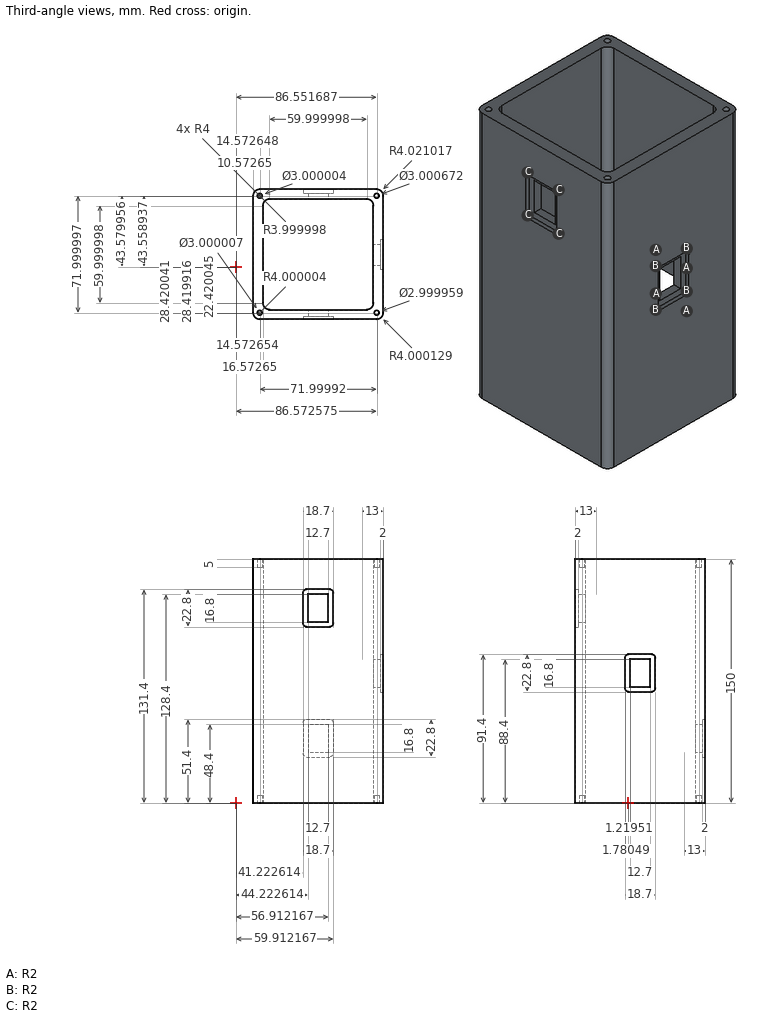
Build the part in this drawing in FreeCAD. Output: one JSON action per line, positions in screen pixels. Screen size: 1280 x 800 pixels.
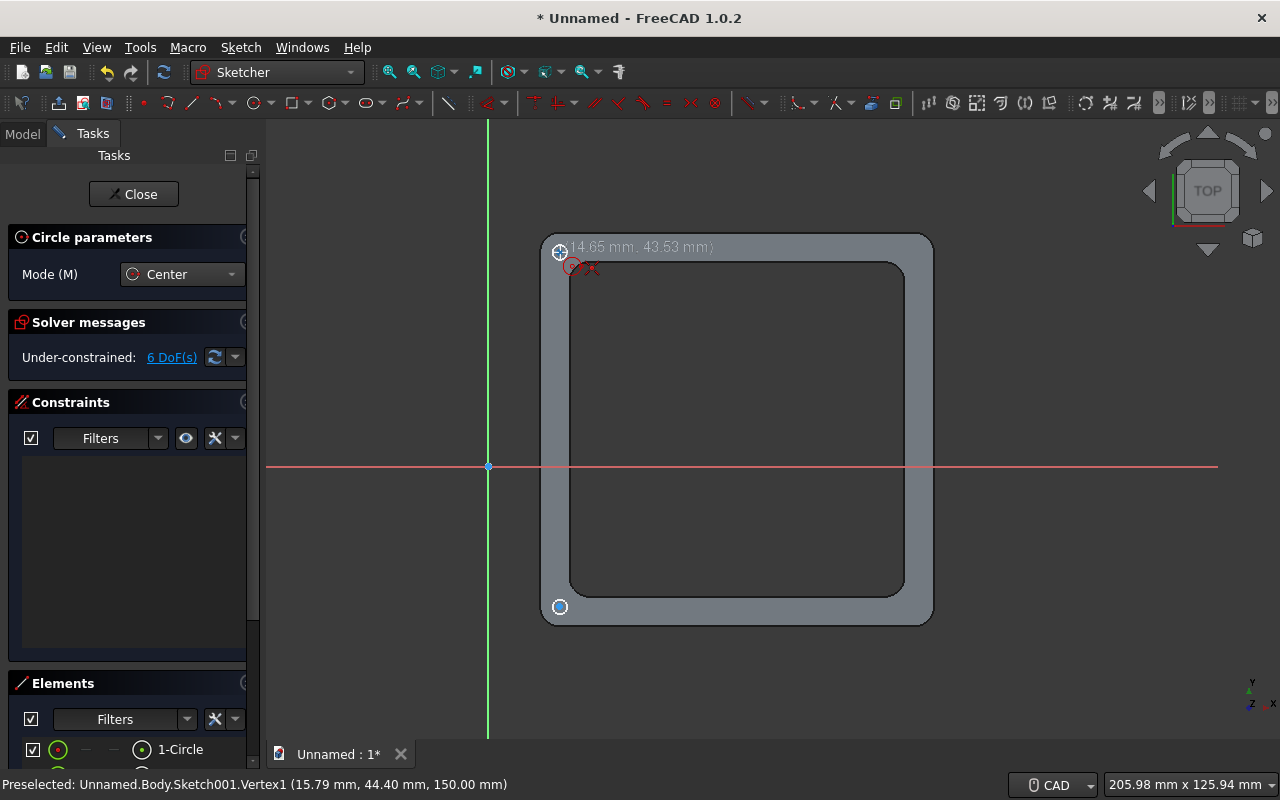
{"action": "scroll", "coordinate": [914, 252], "scroll_direction": "up", "scroll_amount": 6}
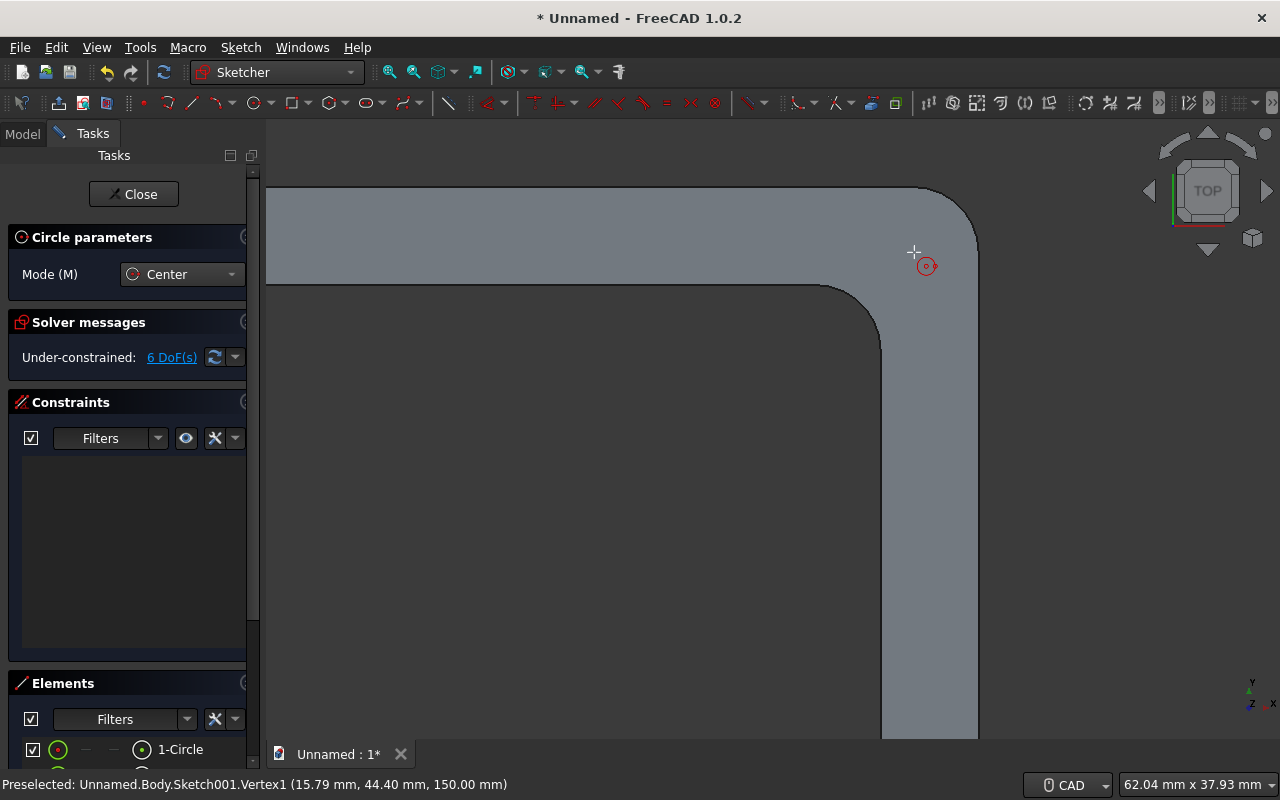
{"action": "left_click", "coordinate": [913, 253]}
{"action": "left_click", "coordinate": [930, 235]}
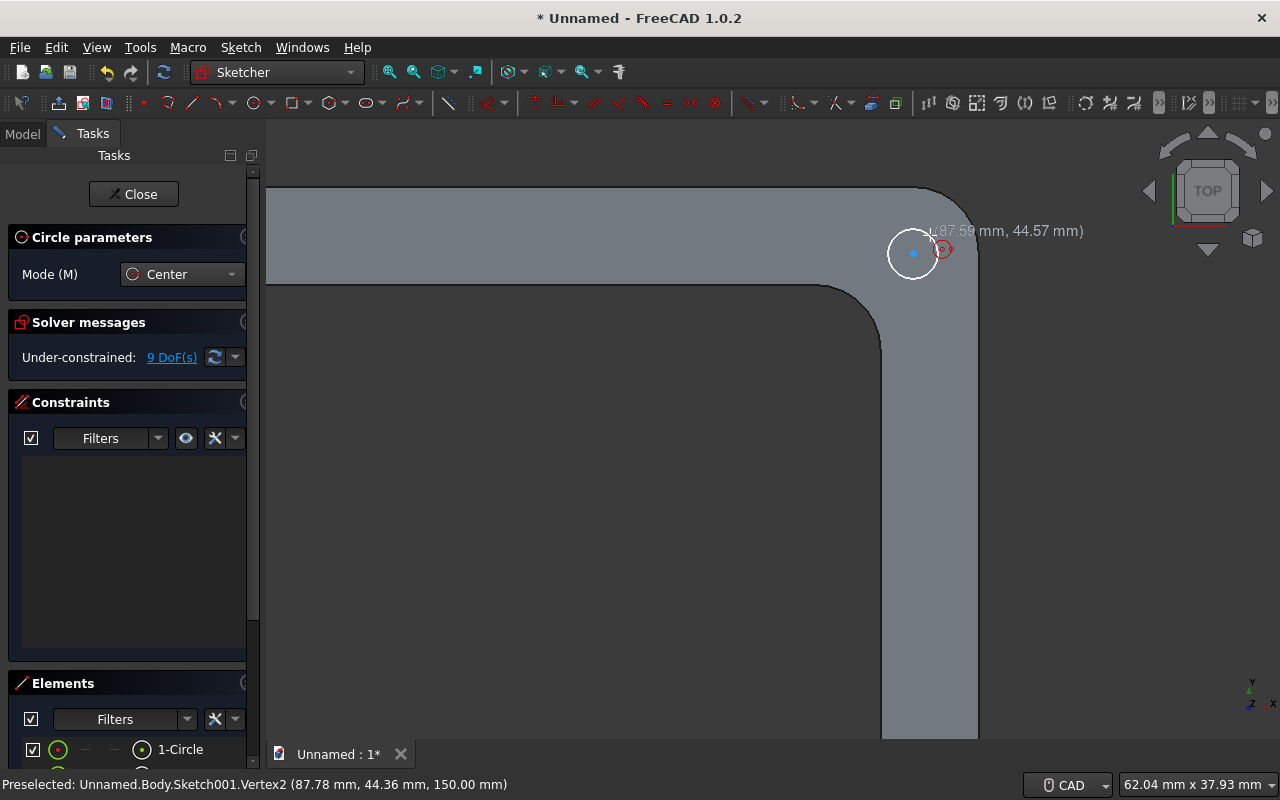
{"action": "scroll", "coordinate": [914, 252], "scroll_direction": "down", "scroll_amount": 6}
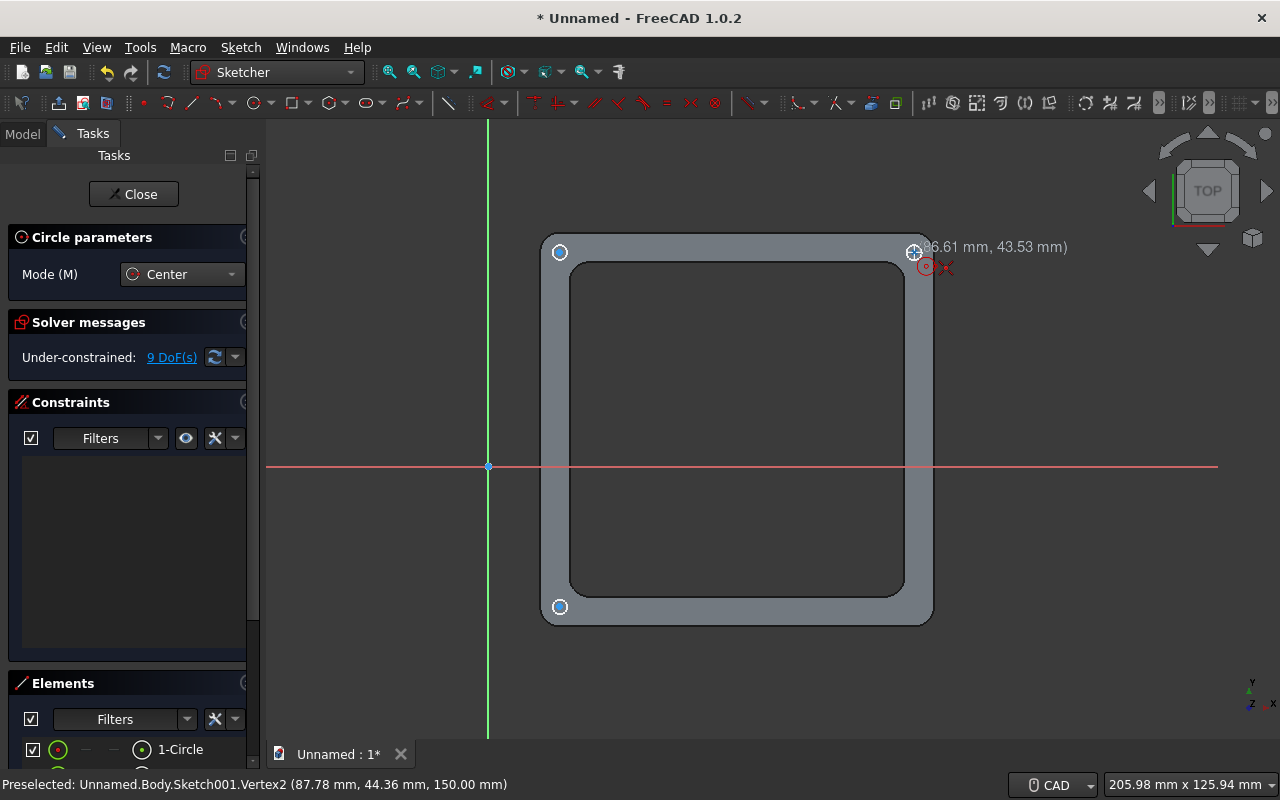
{"action": "scroll", "coordinate": [914, 607], "scroll_direction": "up", "scroll_amount": 6}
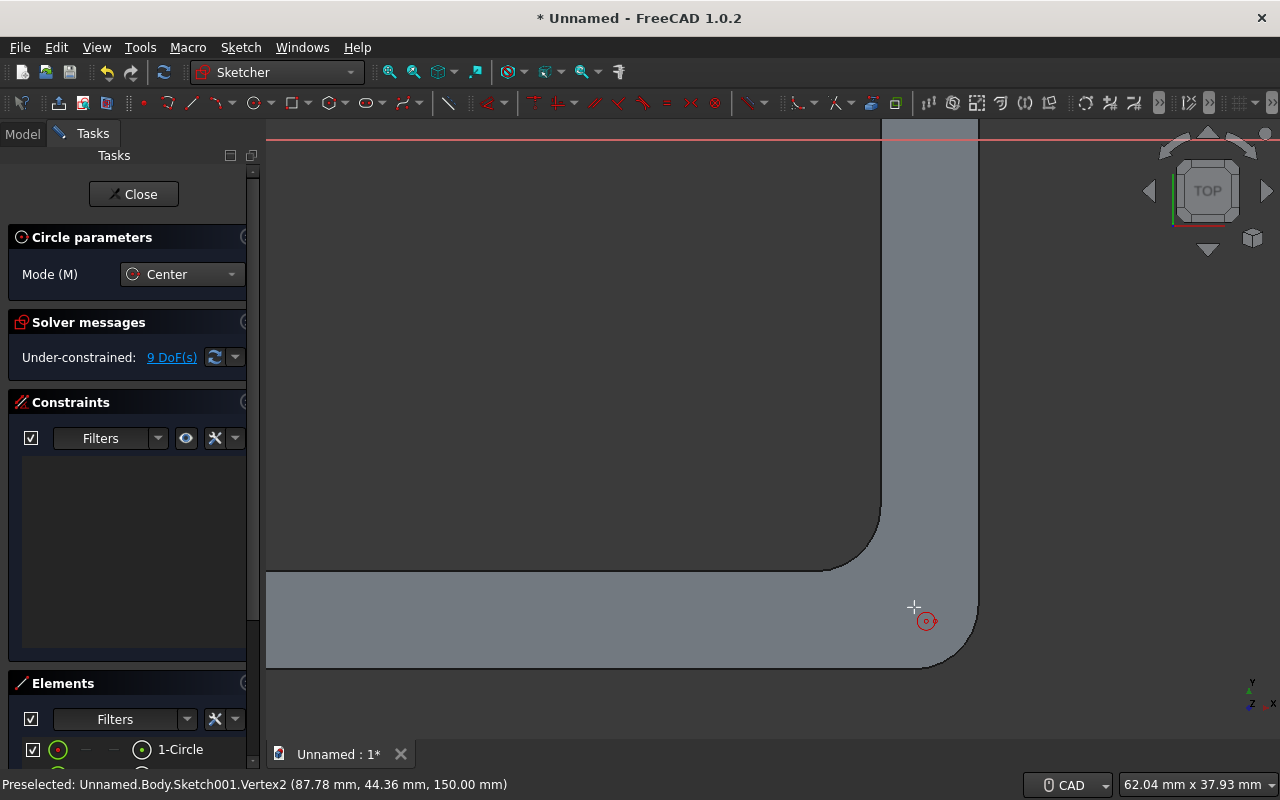
{"action": "left_click", "coordinate": [913, 604]}
{"action": "left_click", "coordinate": [931, 587]}
{"action": "key", "text": "Escape"}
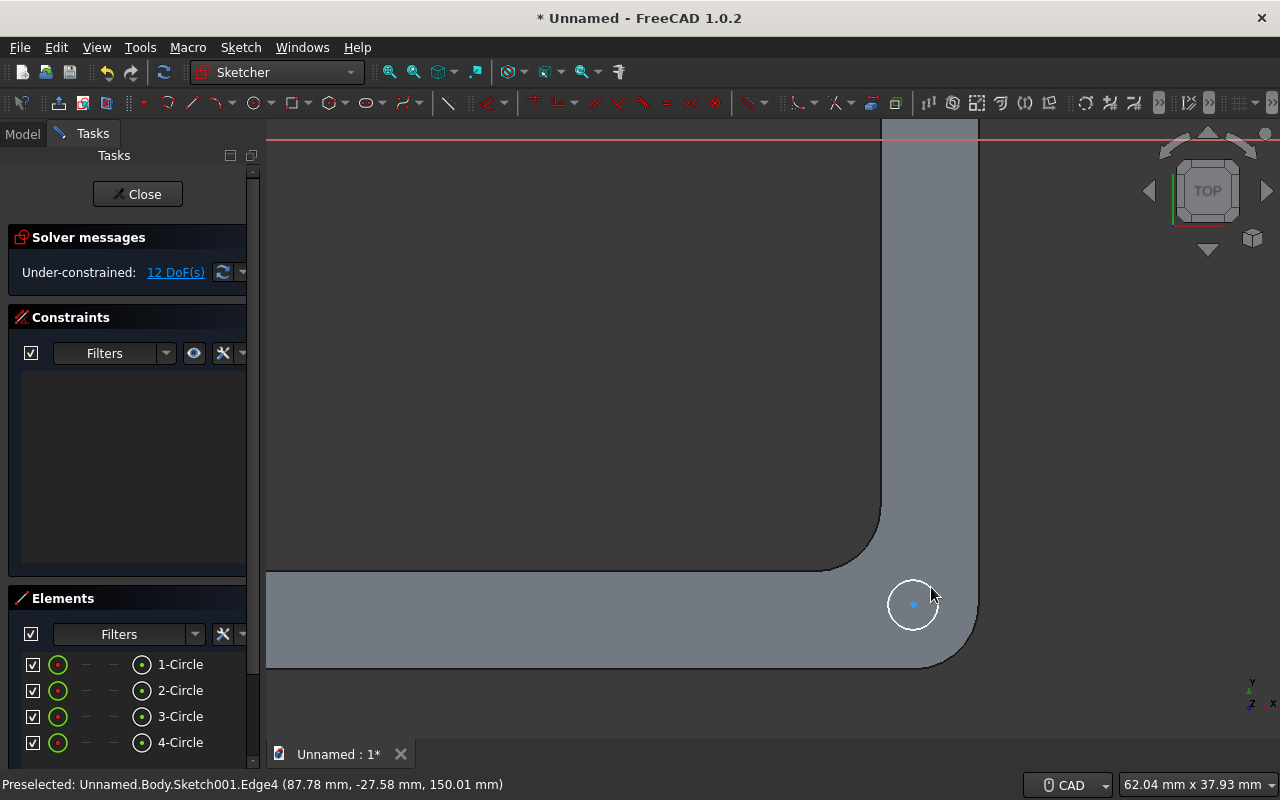
{"action": "left_click", "coordinate": [488, 104]}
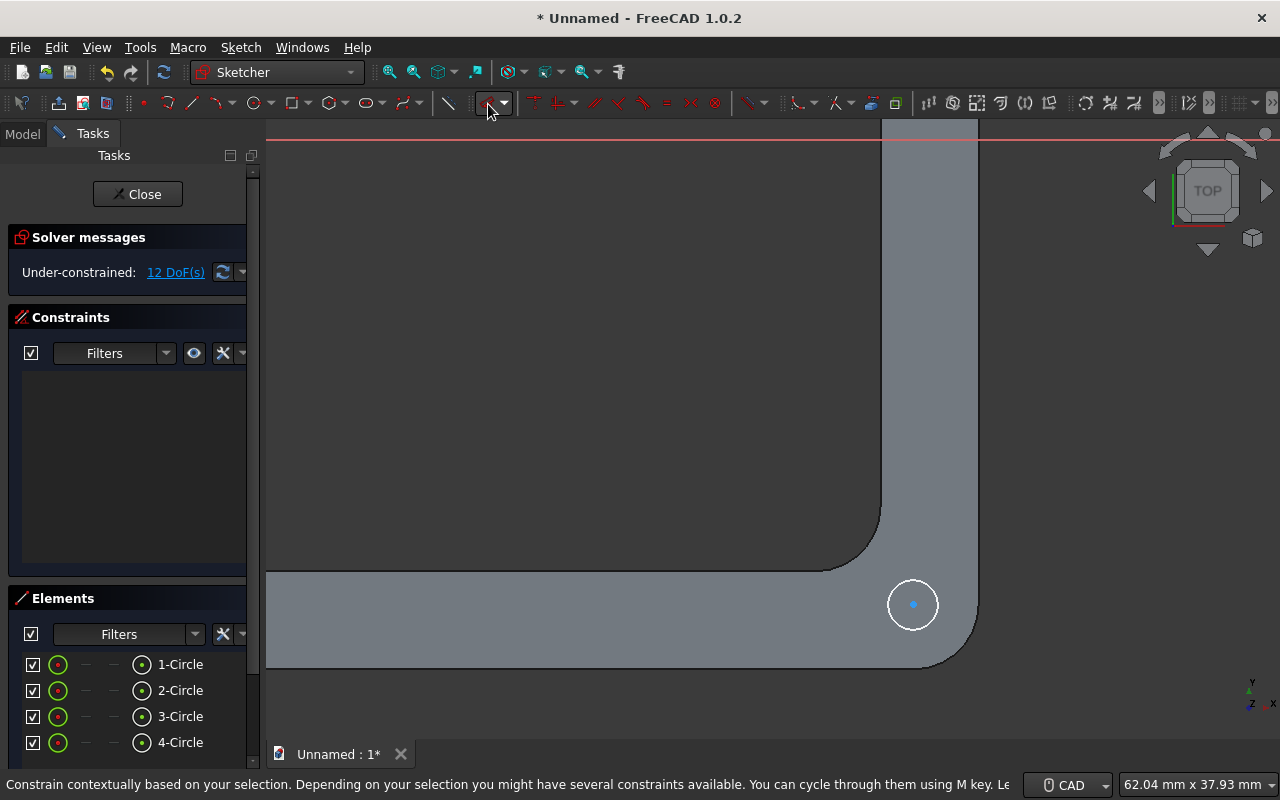
{"action": "scroll", "coordinate": [914, 607], "scroll_direction": "down", "scroll_amount": 6}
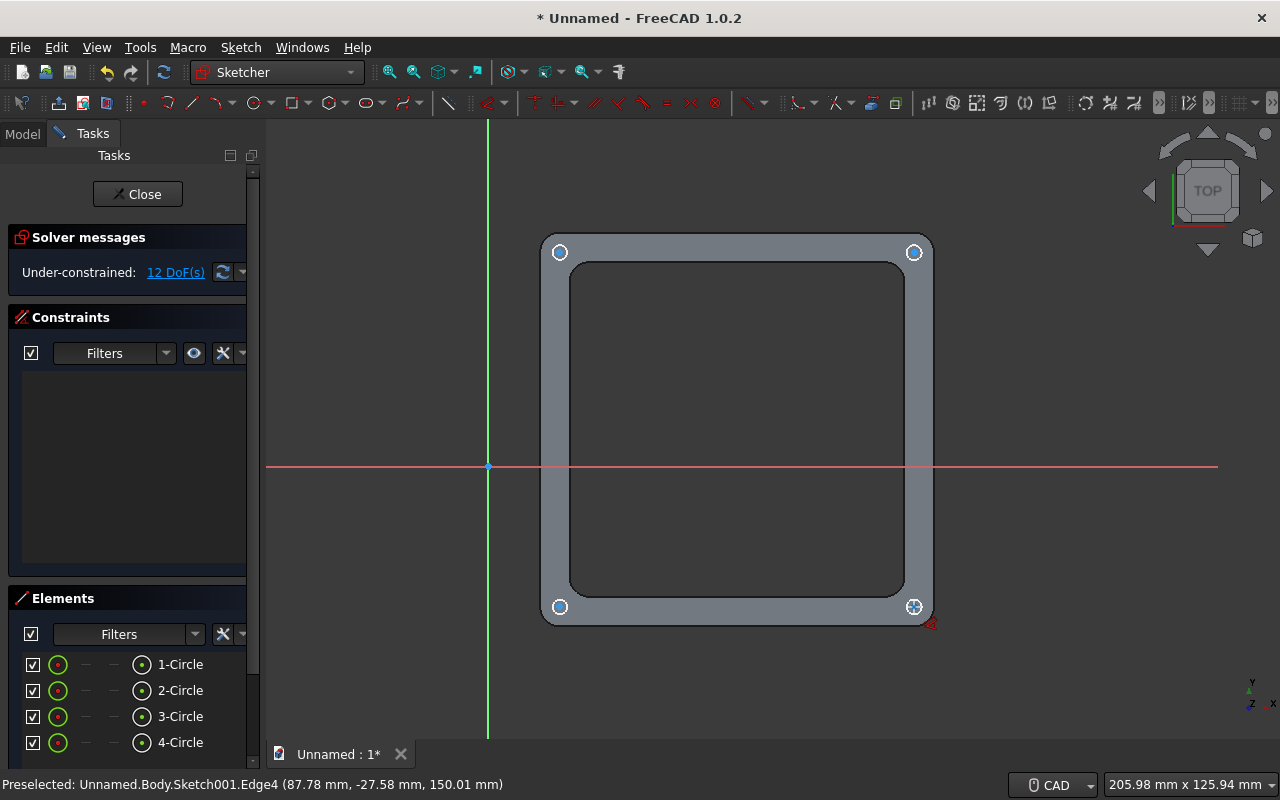
{"action": "scroll", "coordinate": [565, 602], "scroll_direction": "up", "scroll_amount": 5}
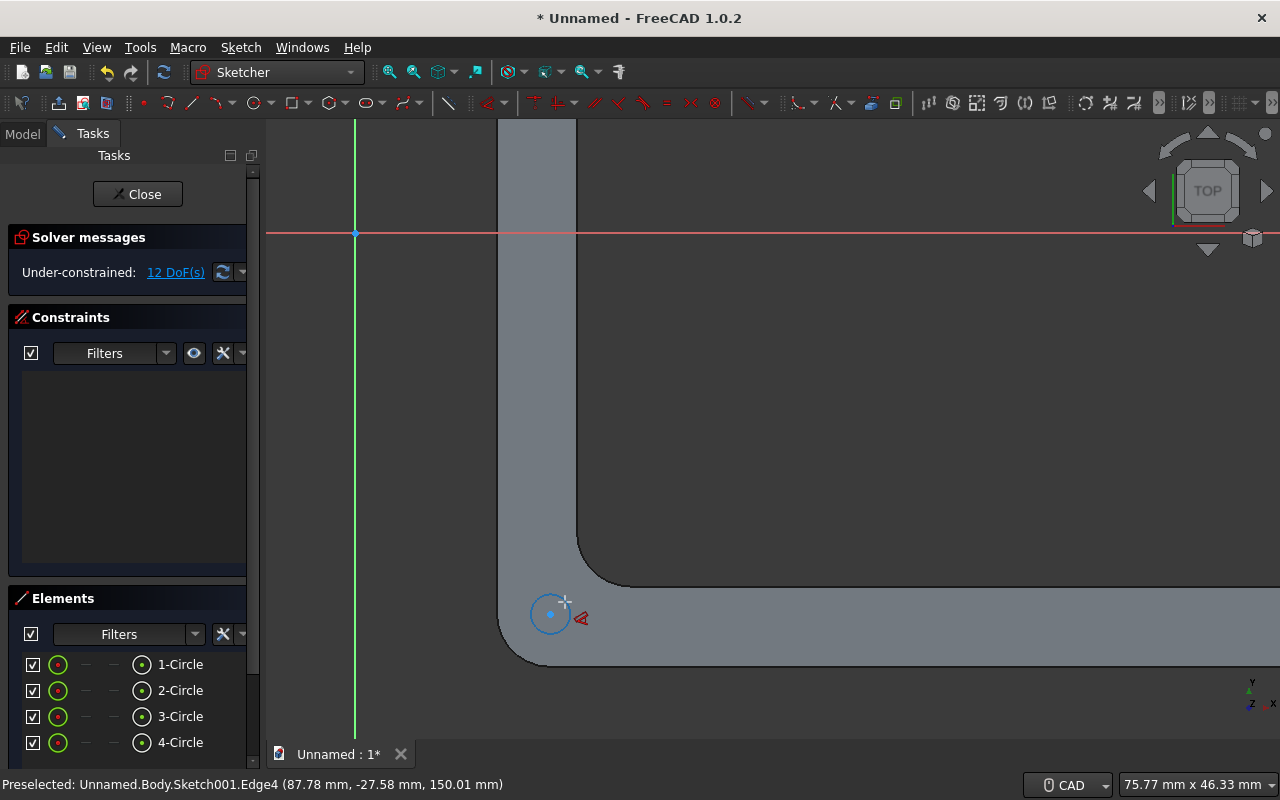
{"action": "left_click", "coordinate": [565, 600]}
{"action": "left_click", "coordinate": [588, 578]}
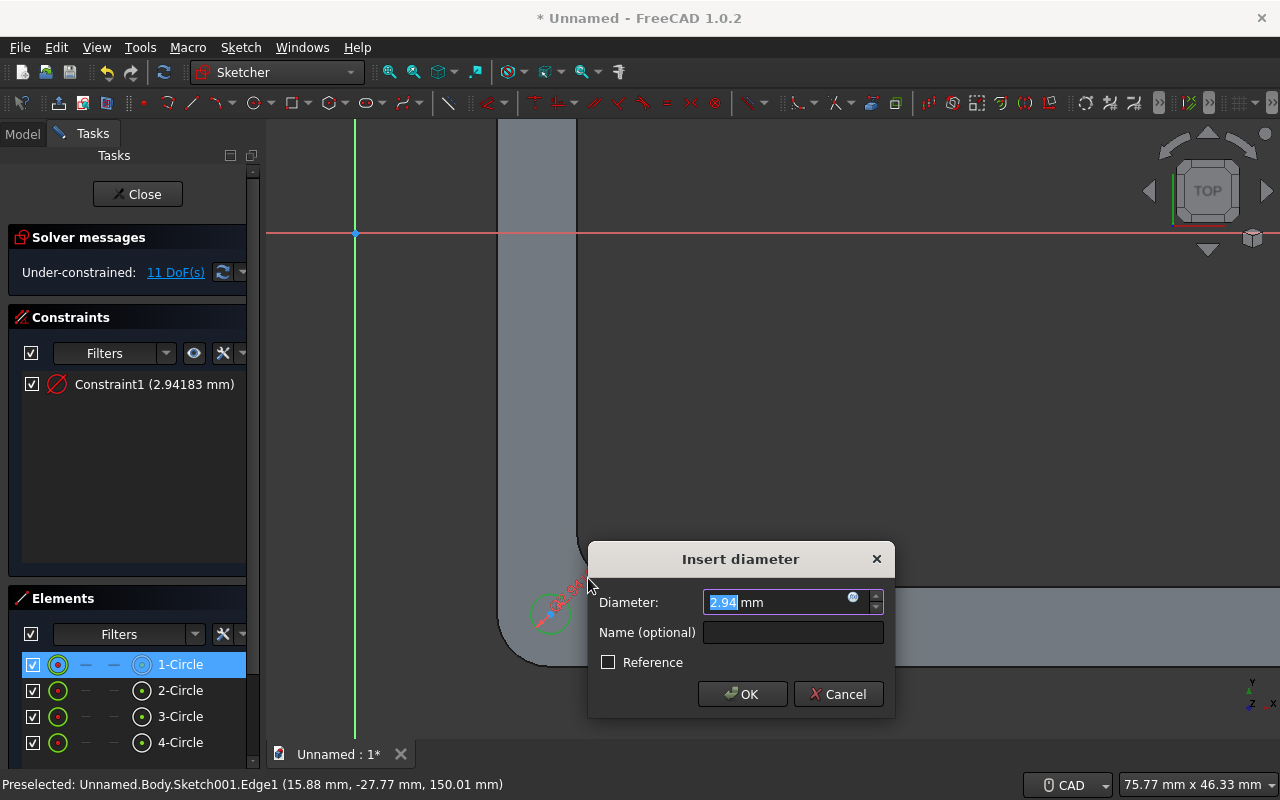
{"action": "type", "text": "3.000007"}
{"action": "key", "text": "Return"}